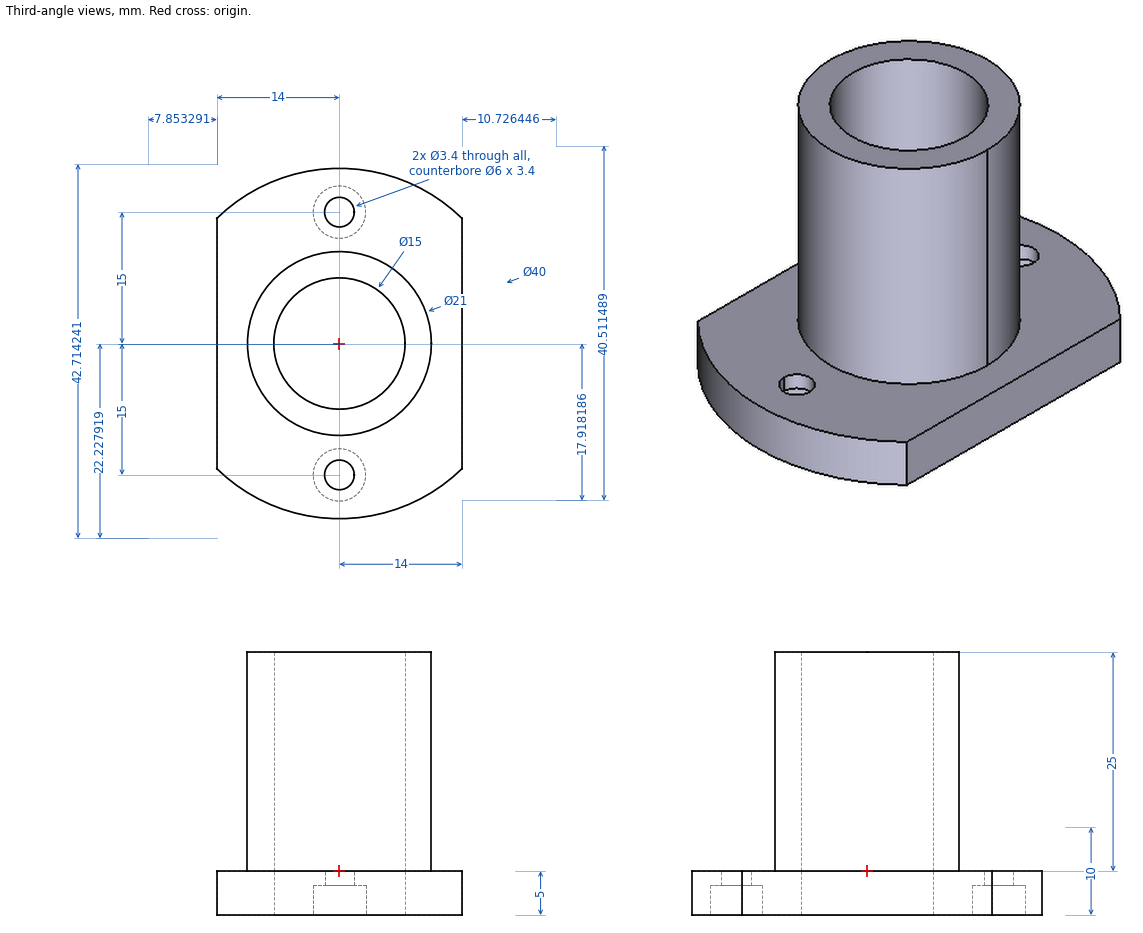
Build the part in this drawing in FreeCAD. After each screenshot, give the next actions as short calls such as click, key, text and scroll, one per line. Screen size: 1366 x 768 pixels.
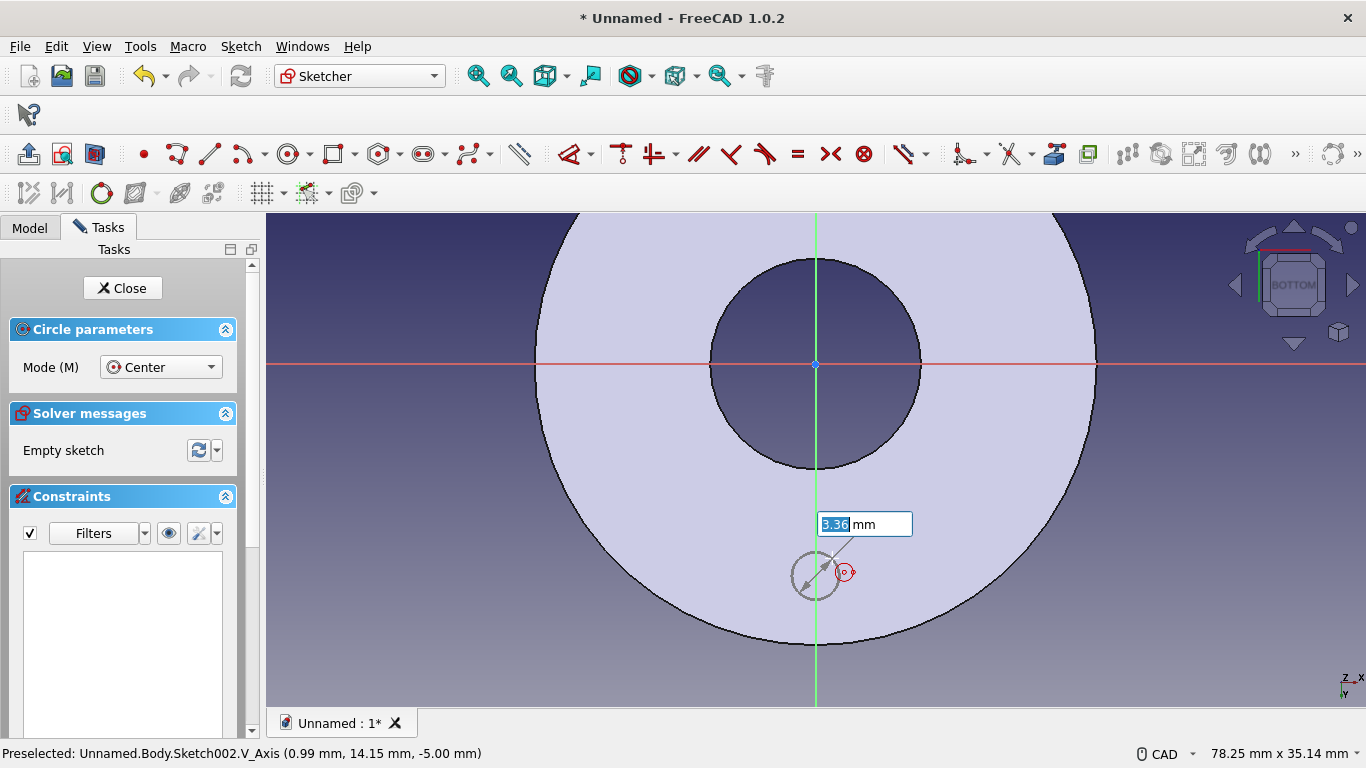
text(3.4)
key(Return)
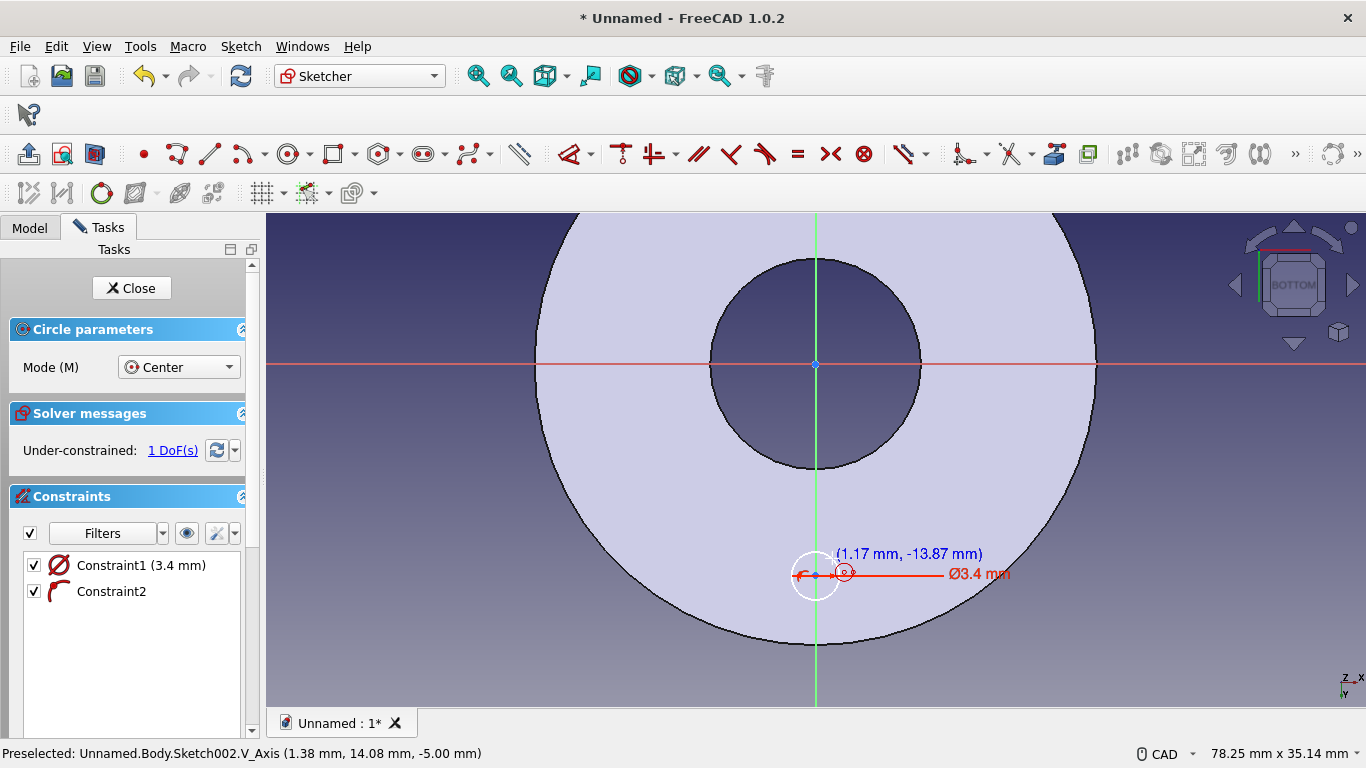
scroll(609, 655, down, 2)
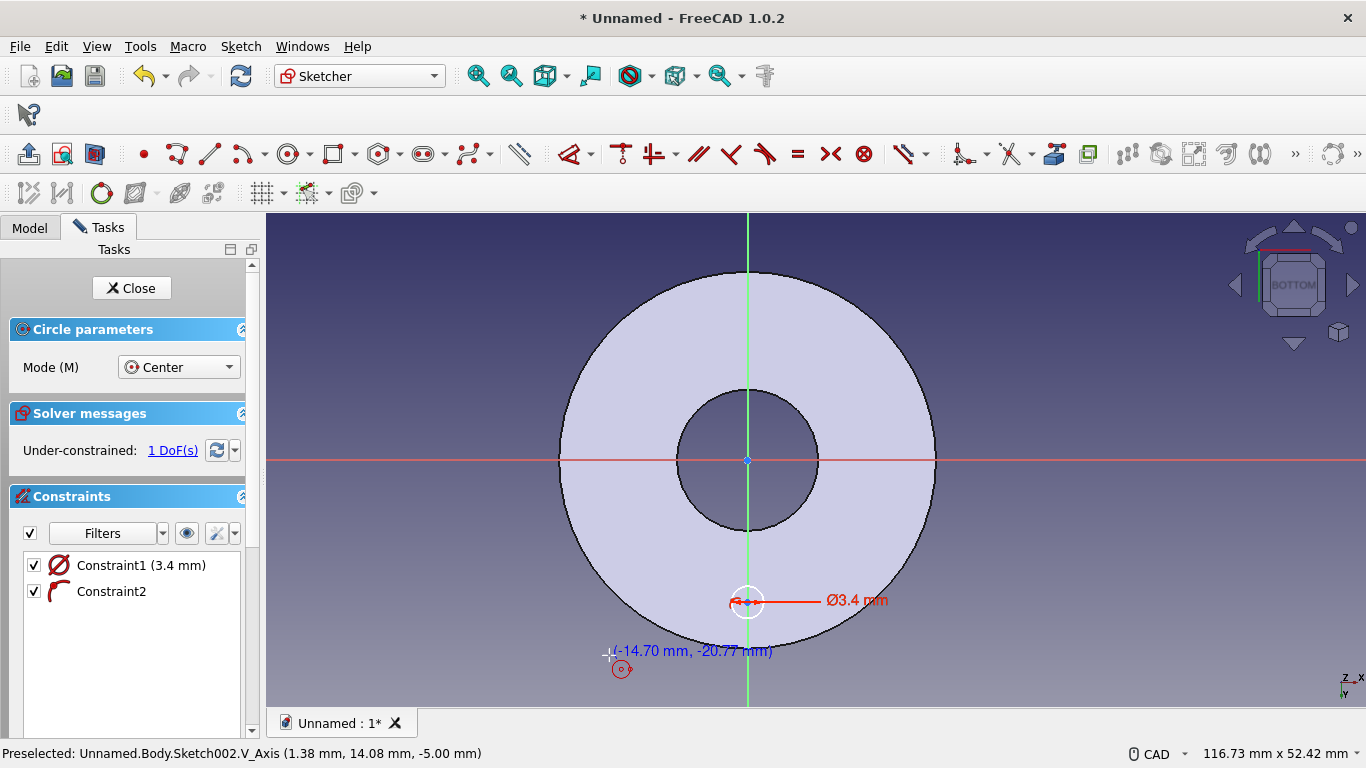
scroll(748, 319, up, 2)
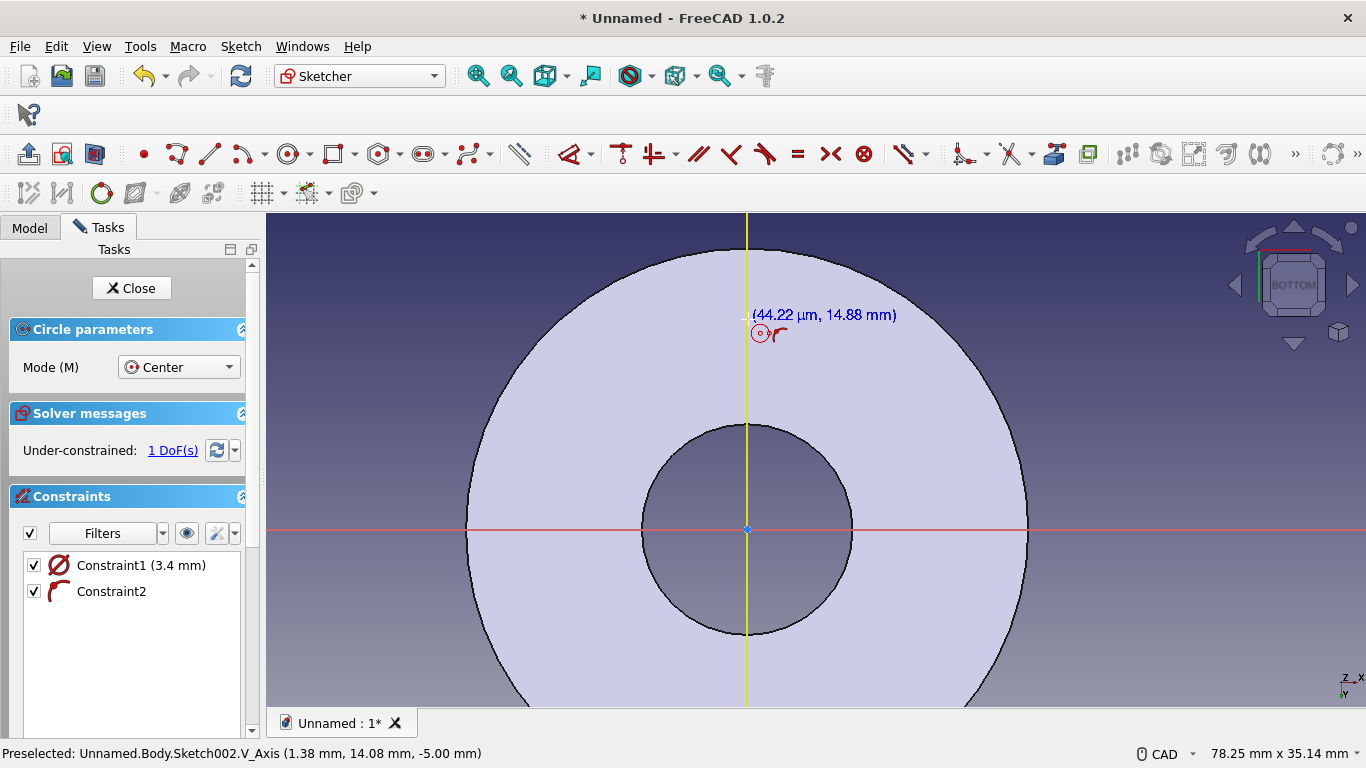
click(747, 319)
move(764, 302)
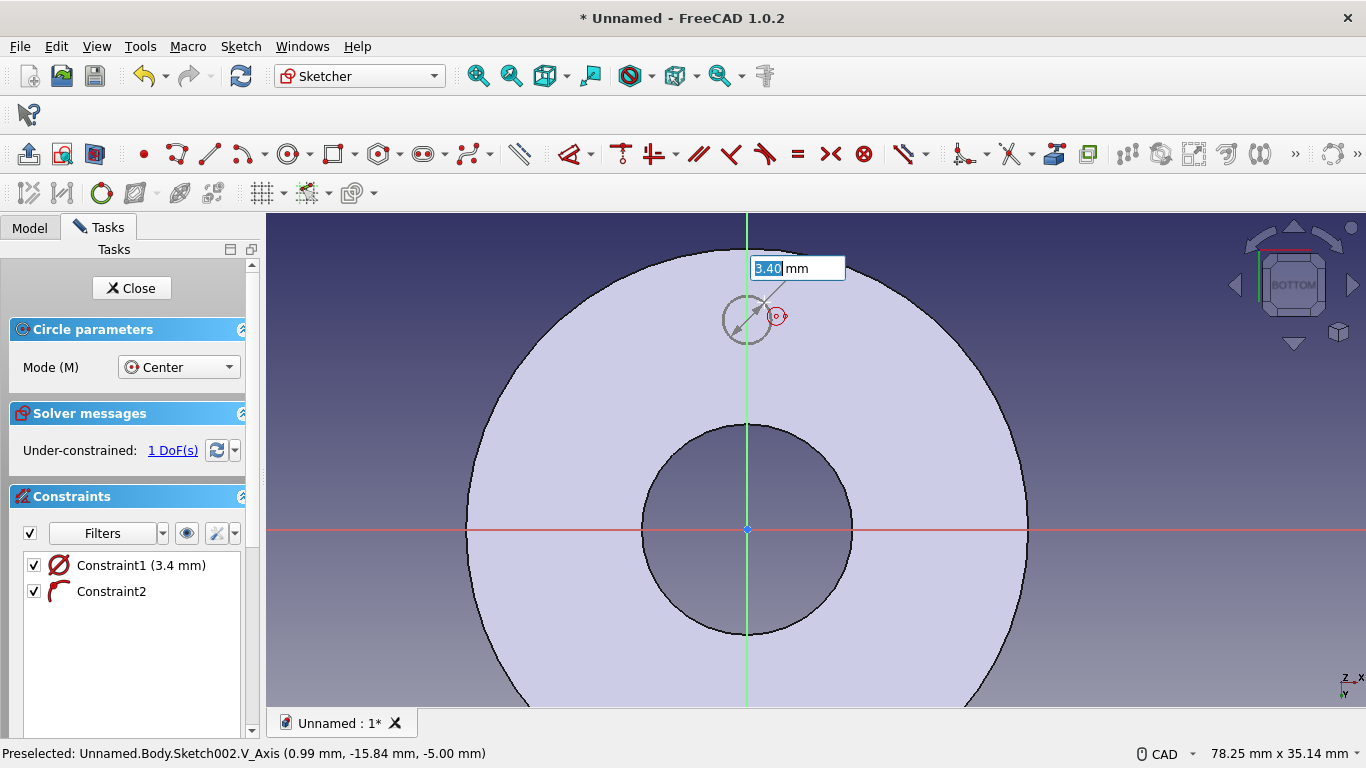
text(3.4)
key(Return)
key(Escape)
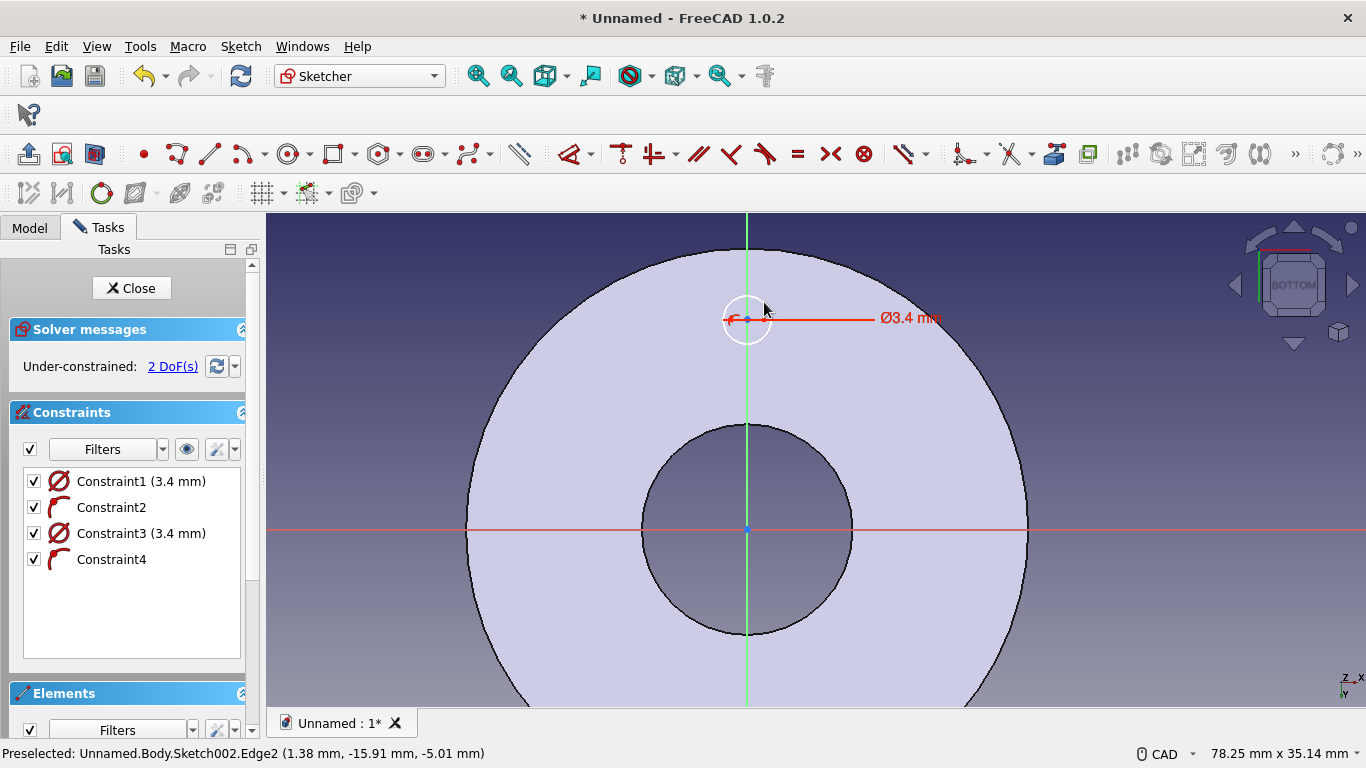
click(568, 154)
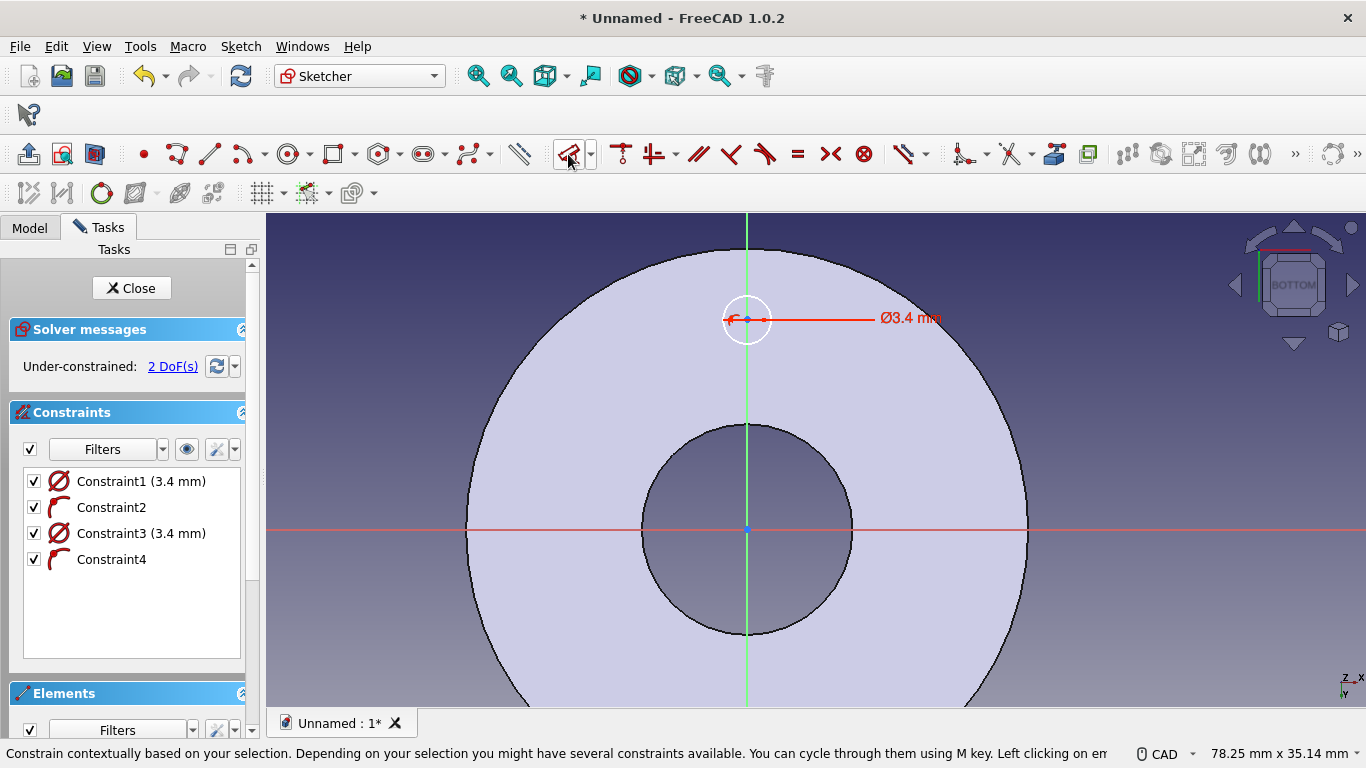
scroll(748, 318, down, 2)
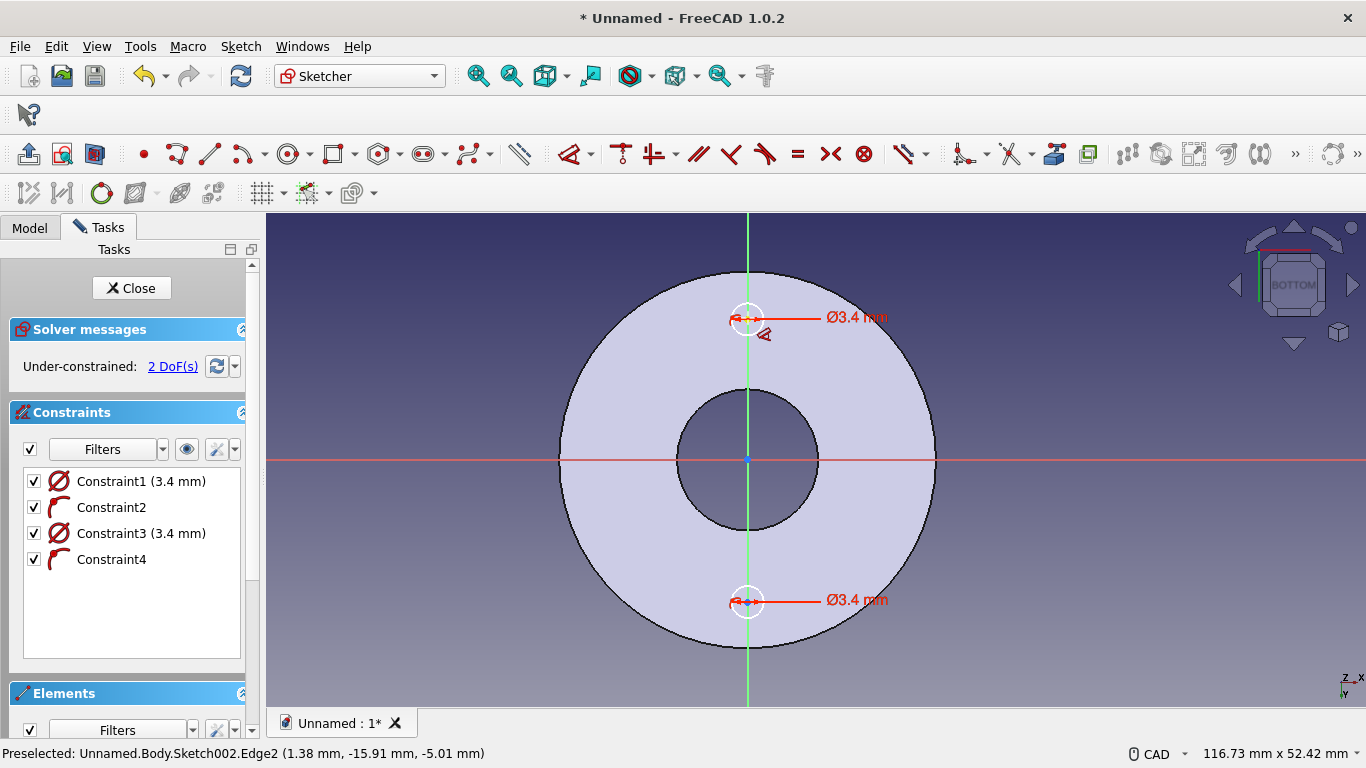
click(748, 602)
click(782, 531)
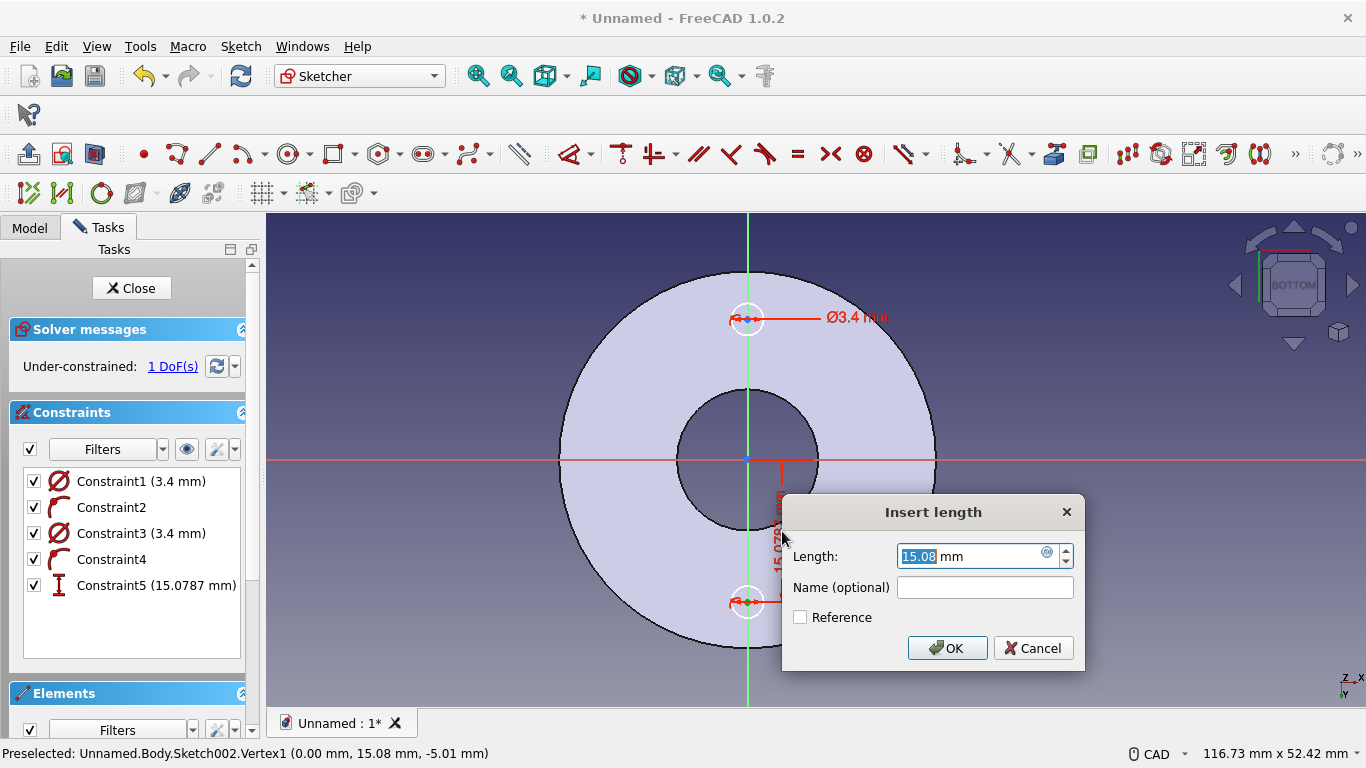
text(15)
key(Return)